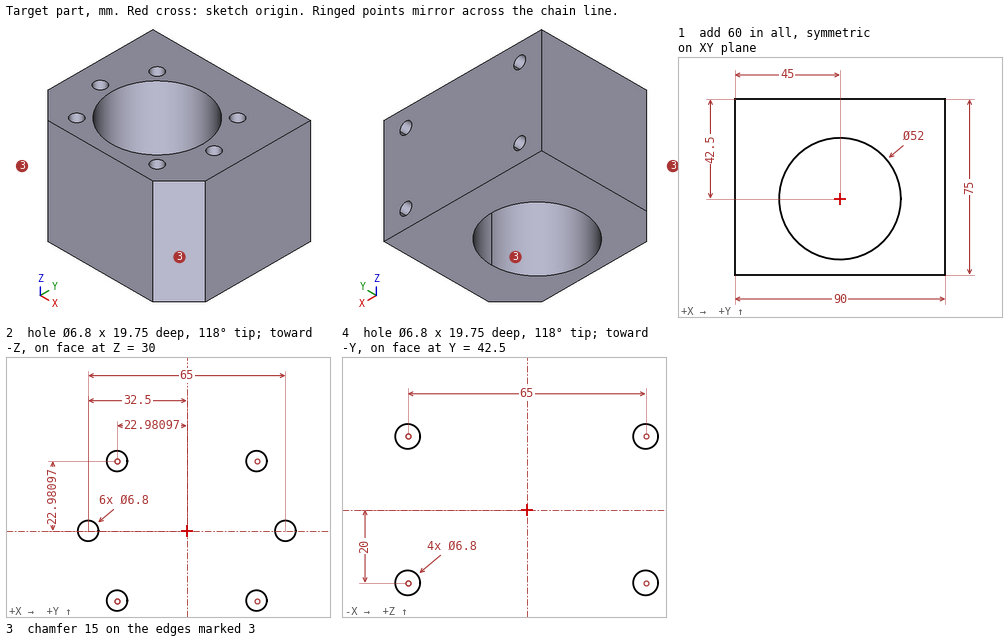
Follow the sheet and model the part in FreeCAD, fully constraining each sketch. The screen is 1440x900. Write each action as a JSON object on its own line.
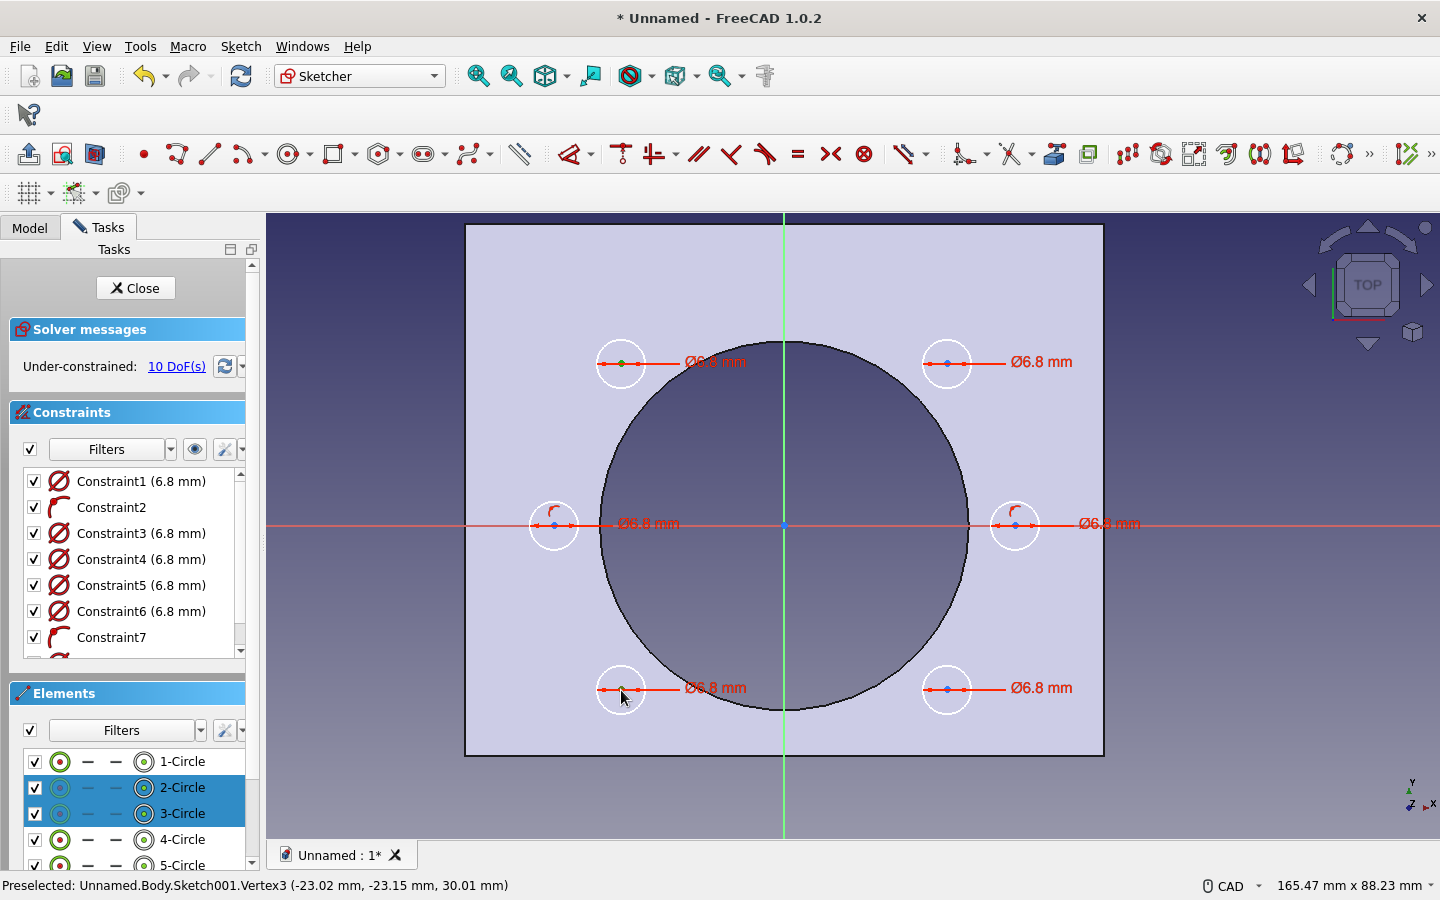
{"action": "left_click", "coordinate": [364, 526]}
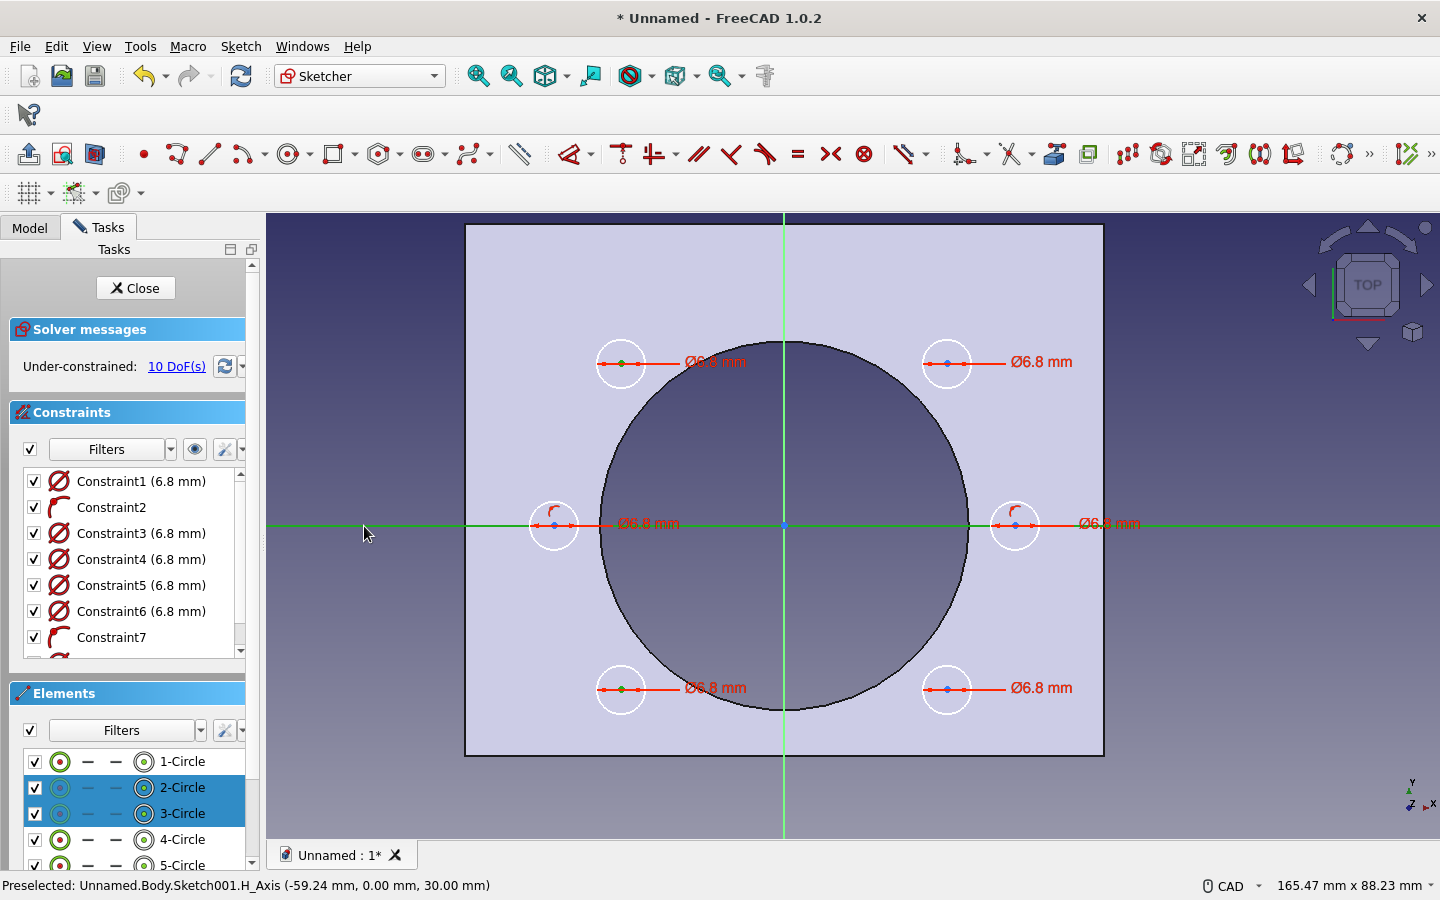
{"action": "left_click", "coordinate": [831, 154]}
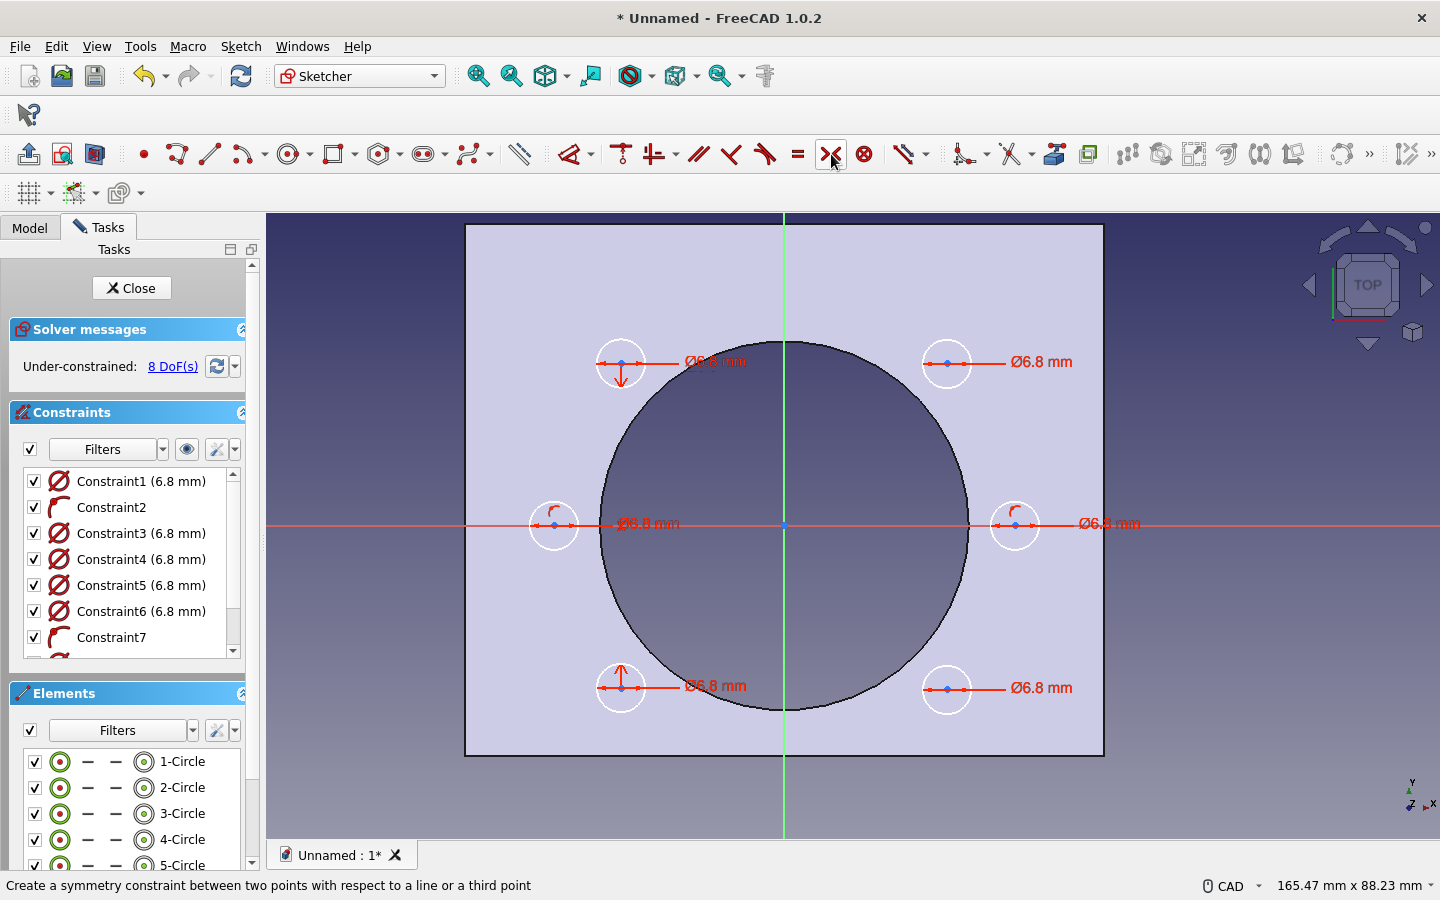
{"action": "left_click", "coordinate": [621, 688]}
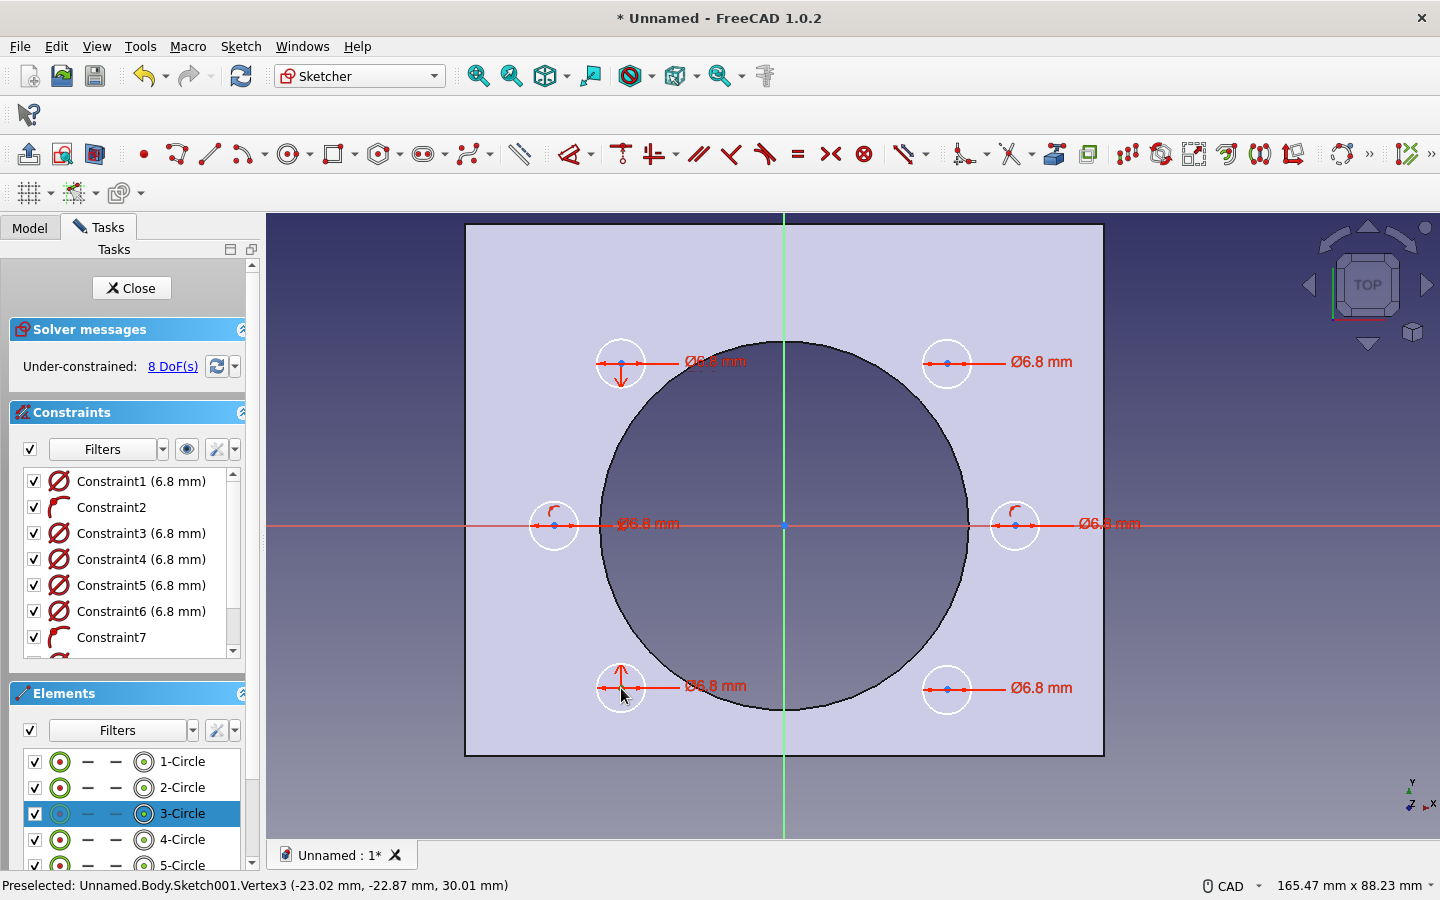
{"action": "left_click", "coordinate": [947, 690]}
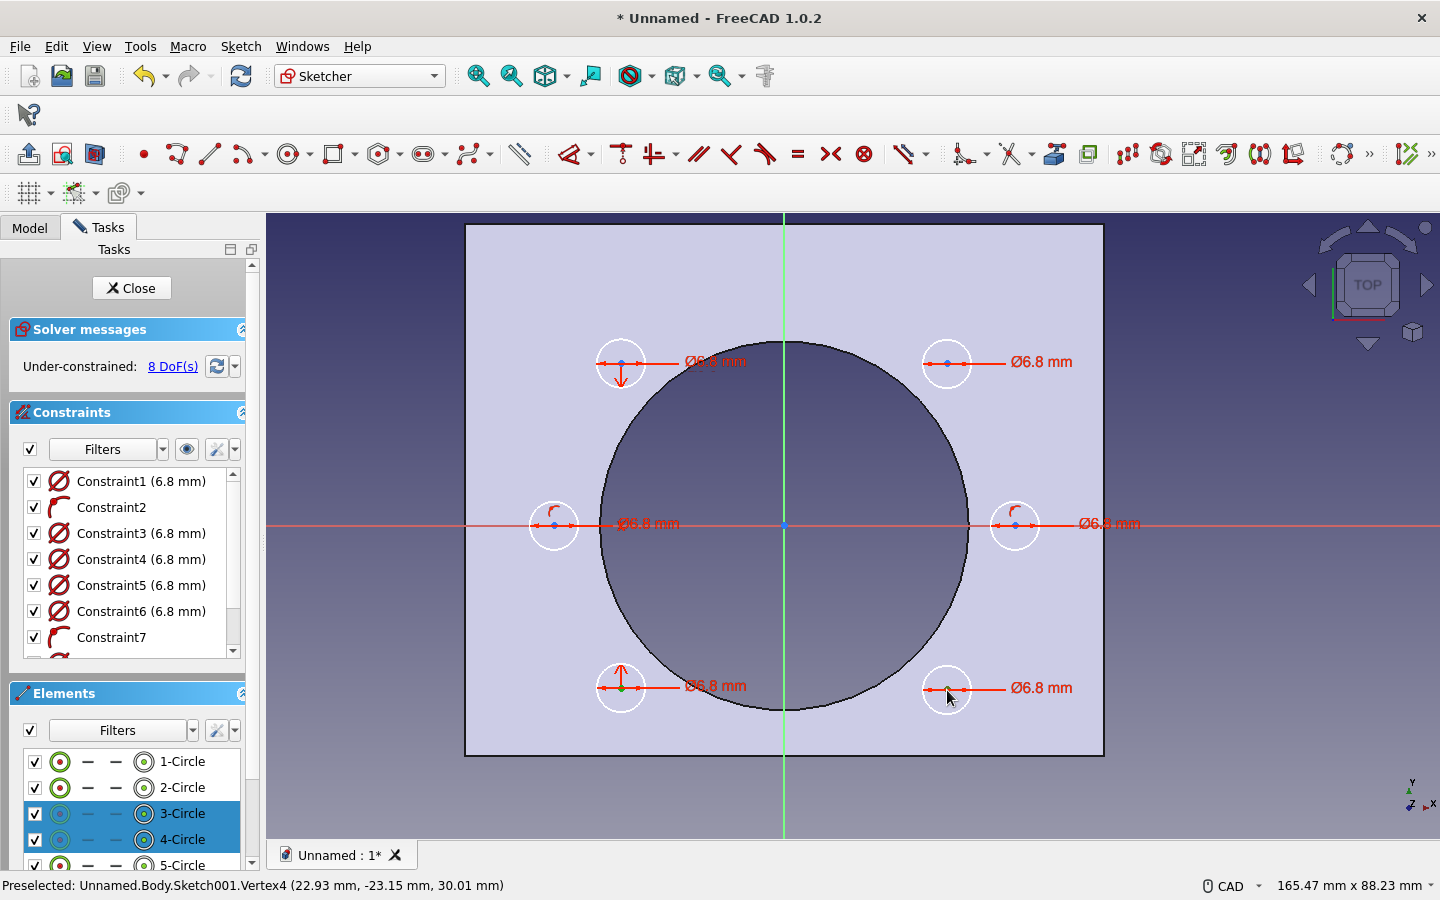
{"action": "left_click", "coordinate": [784, 770]}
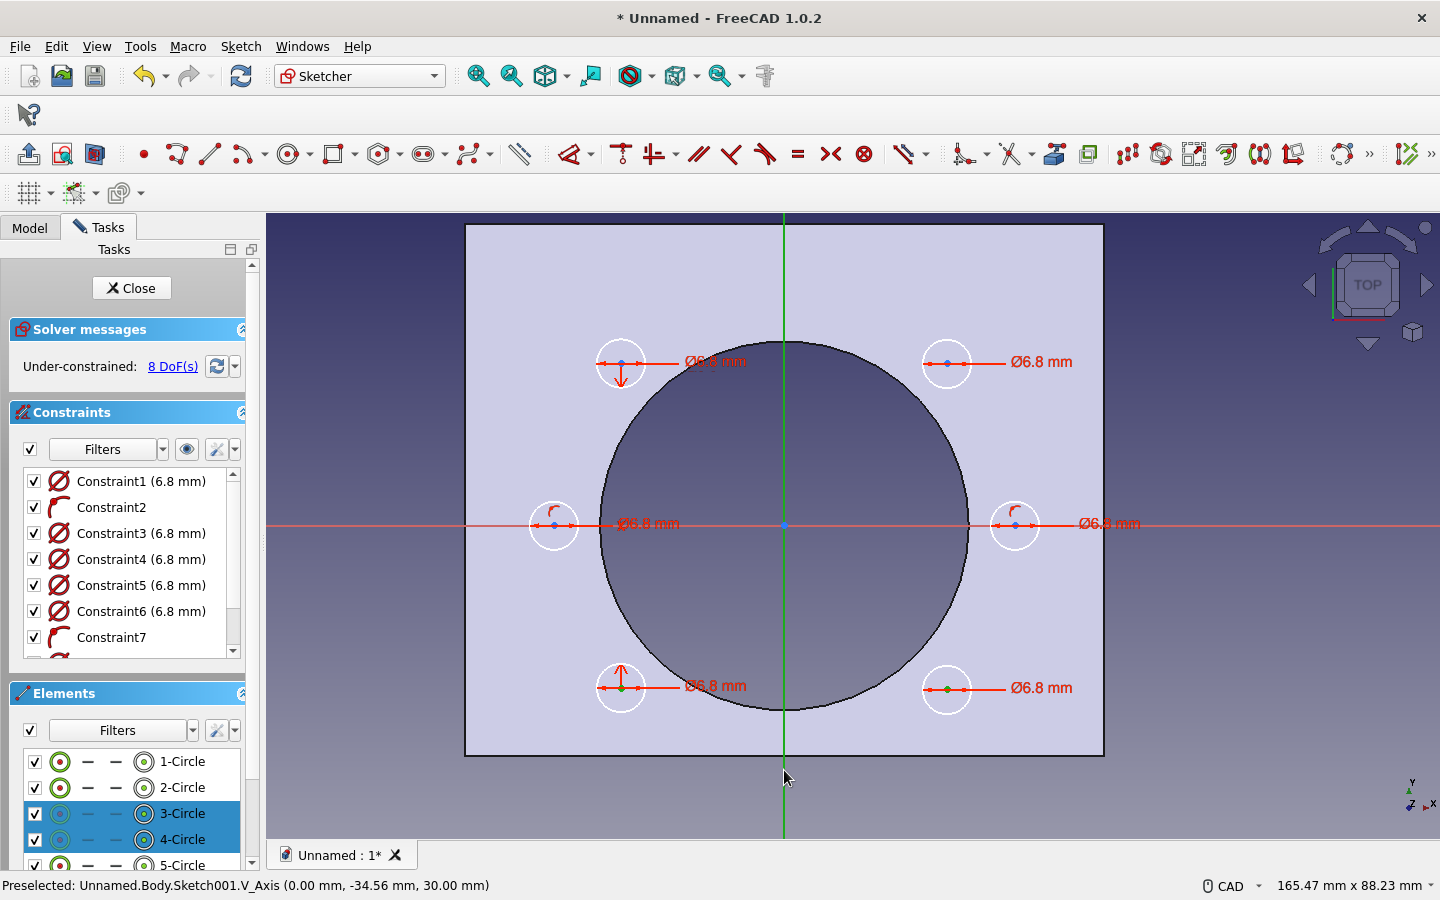
{"action": "key", "text": "s"}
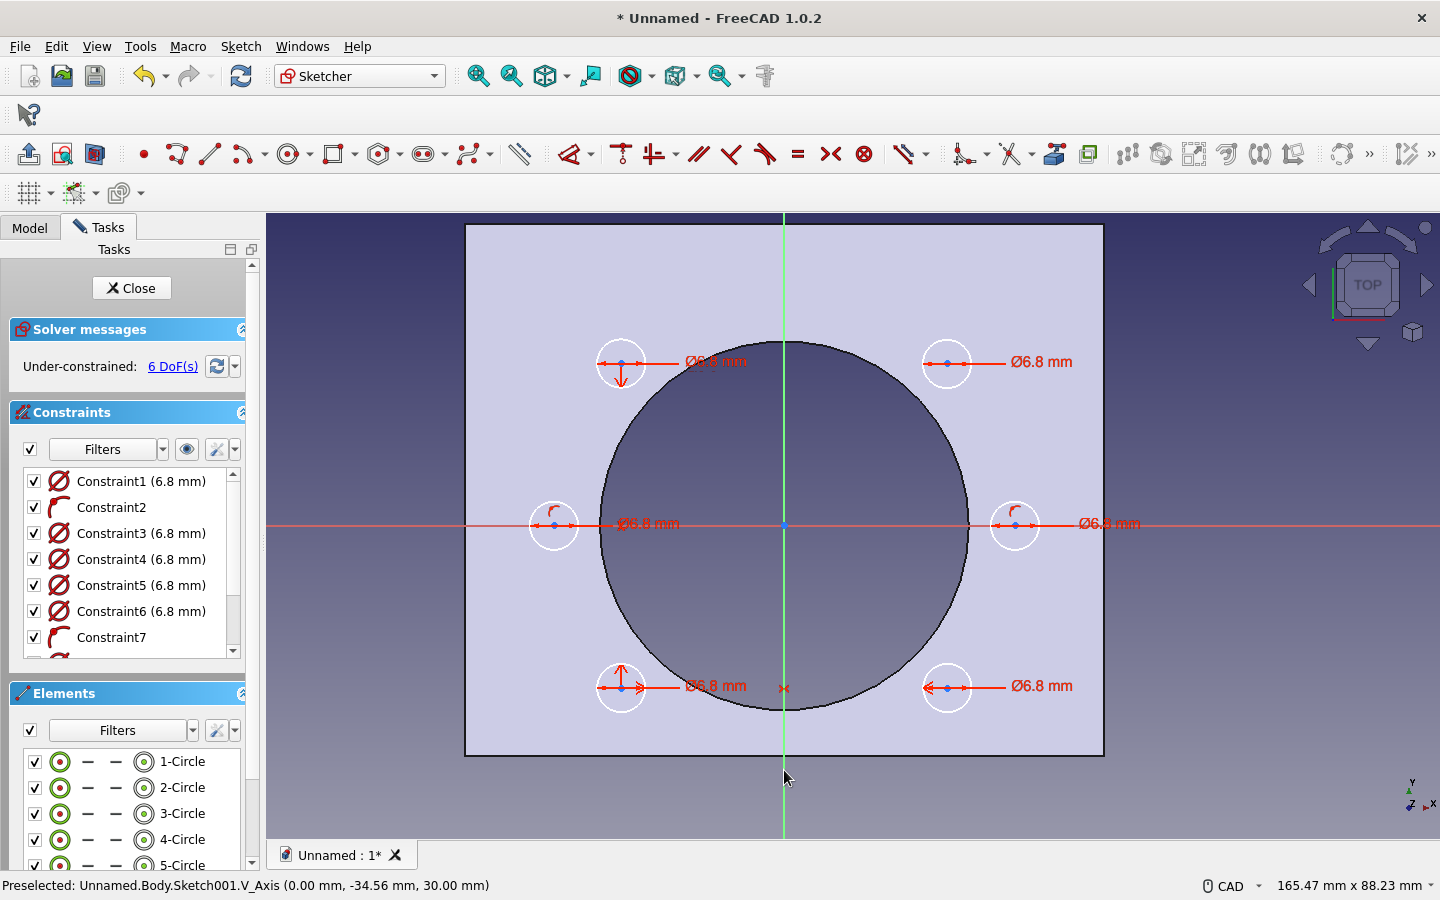
{"action": "left_click", "coordinate": [621, 363]}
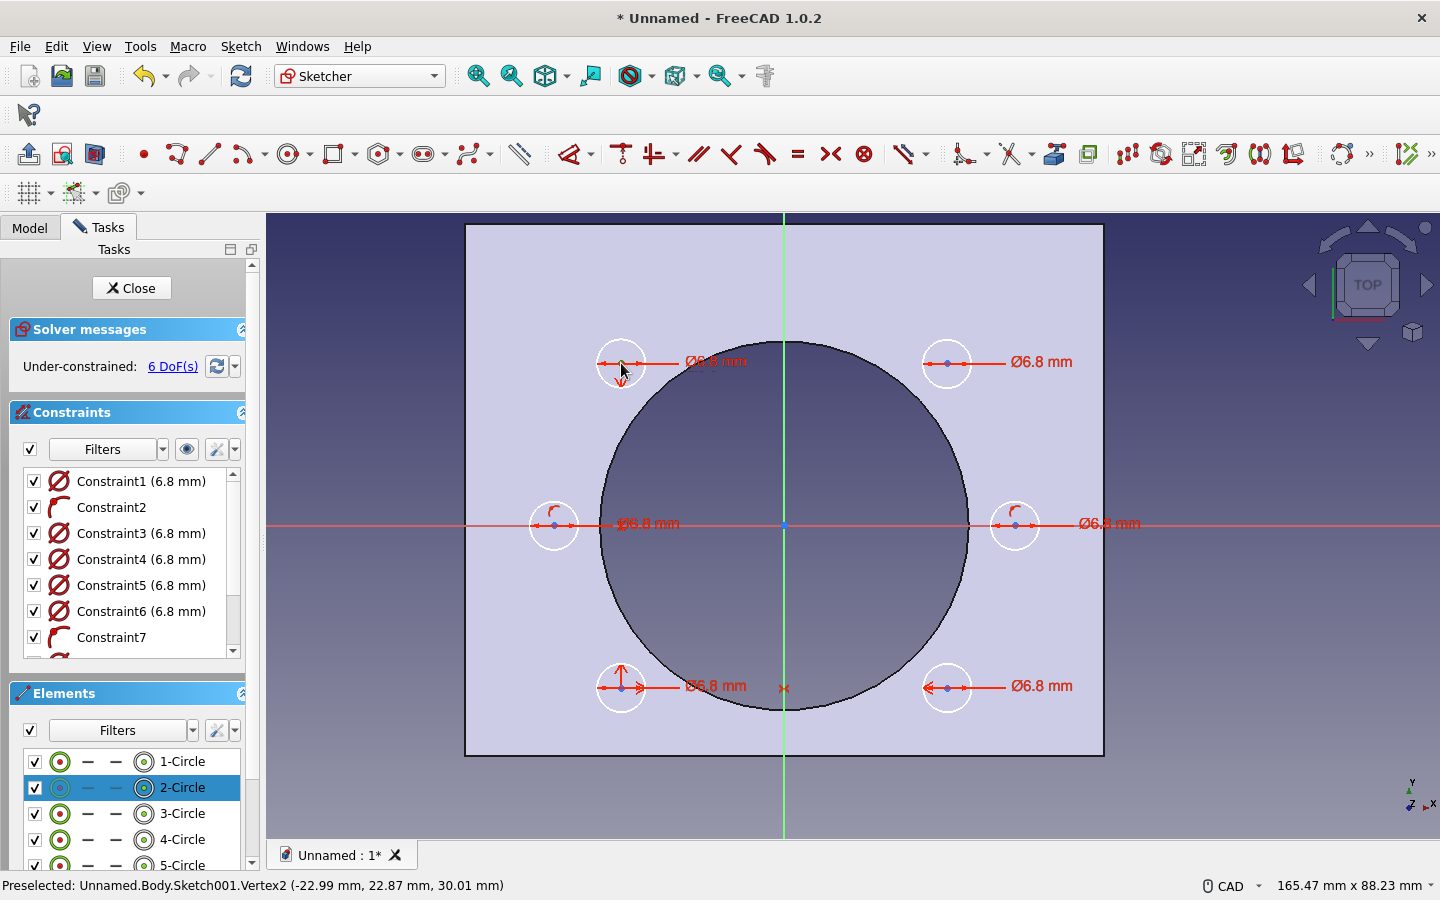
{"action": "left_click", "coordinate": [947, 364]}